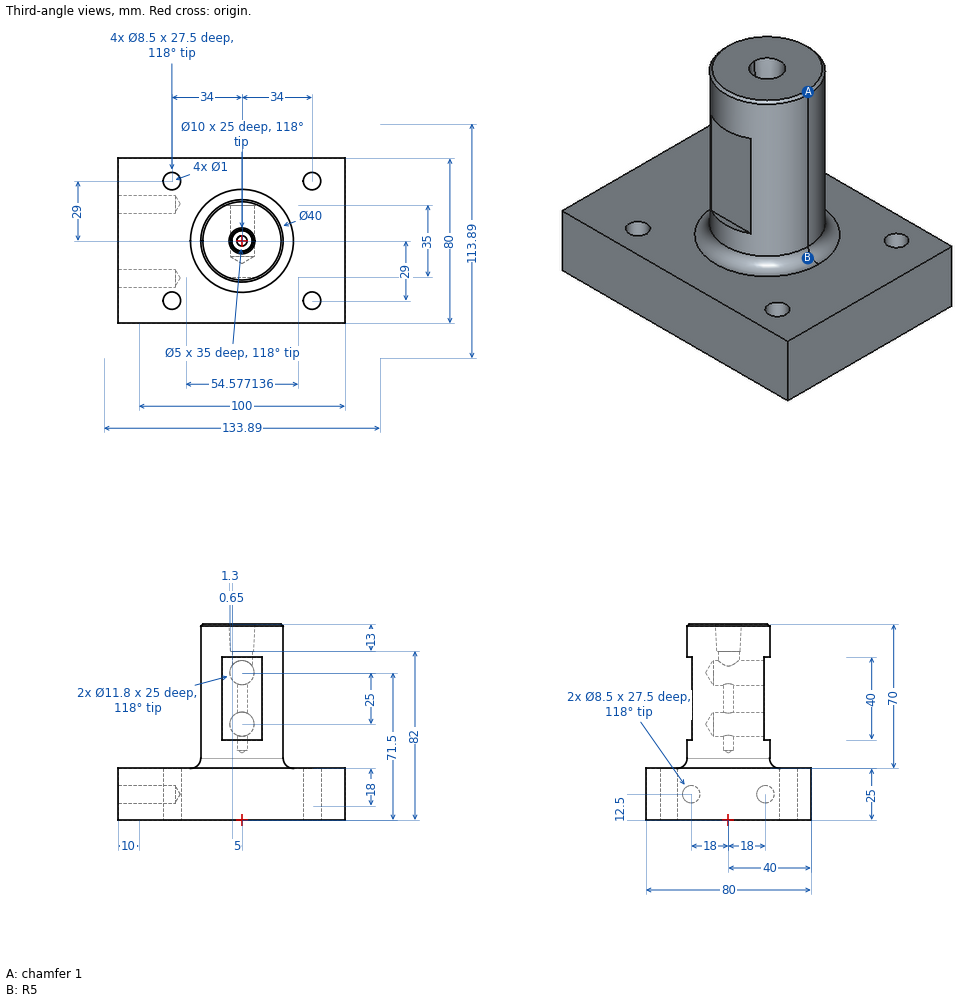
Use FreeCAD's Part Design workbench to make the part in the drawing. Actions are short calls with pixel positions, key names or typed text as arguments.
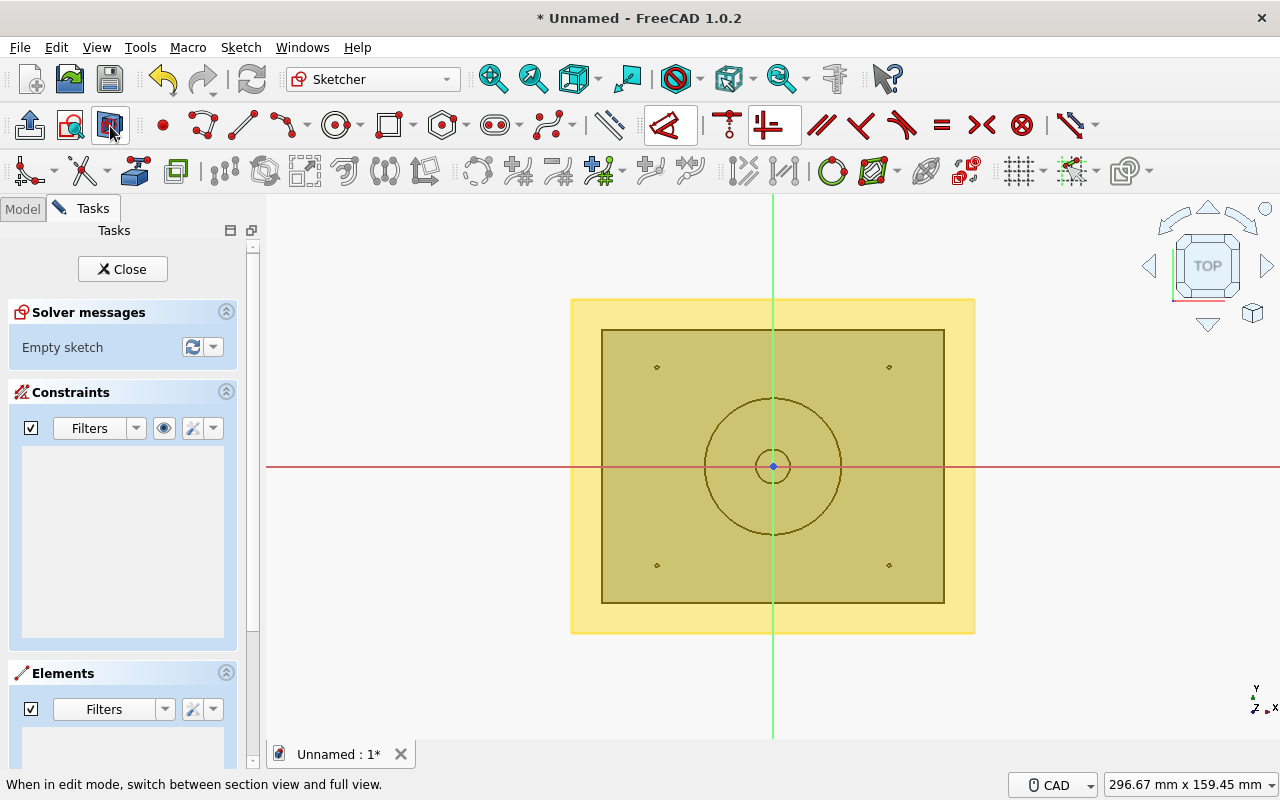
click(416, 126)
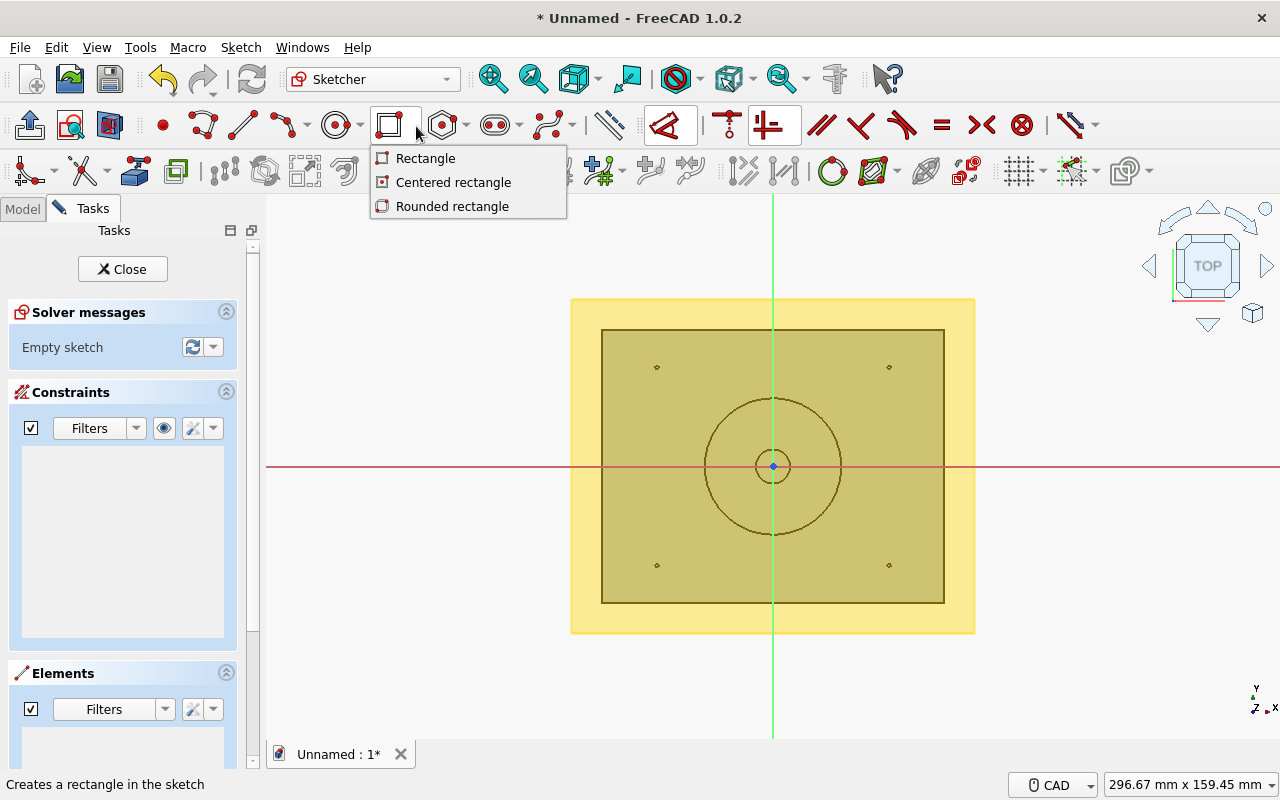
click(468, 182)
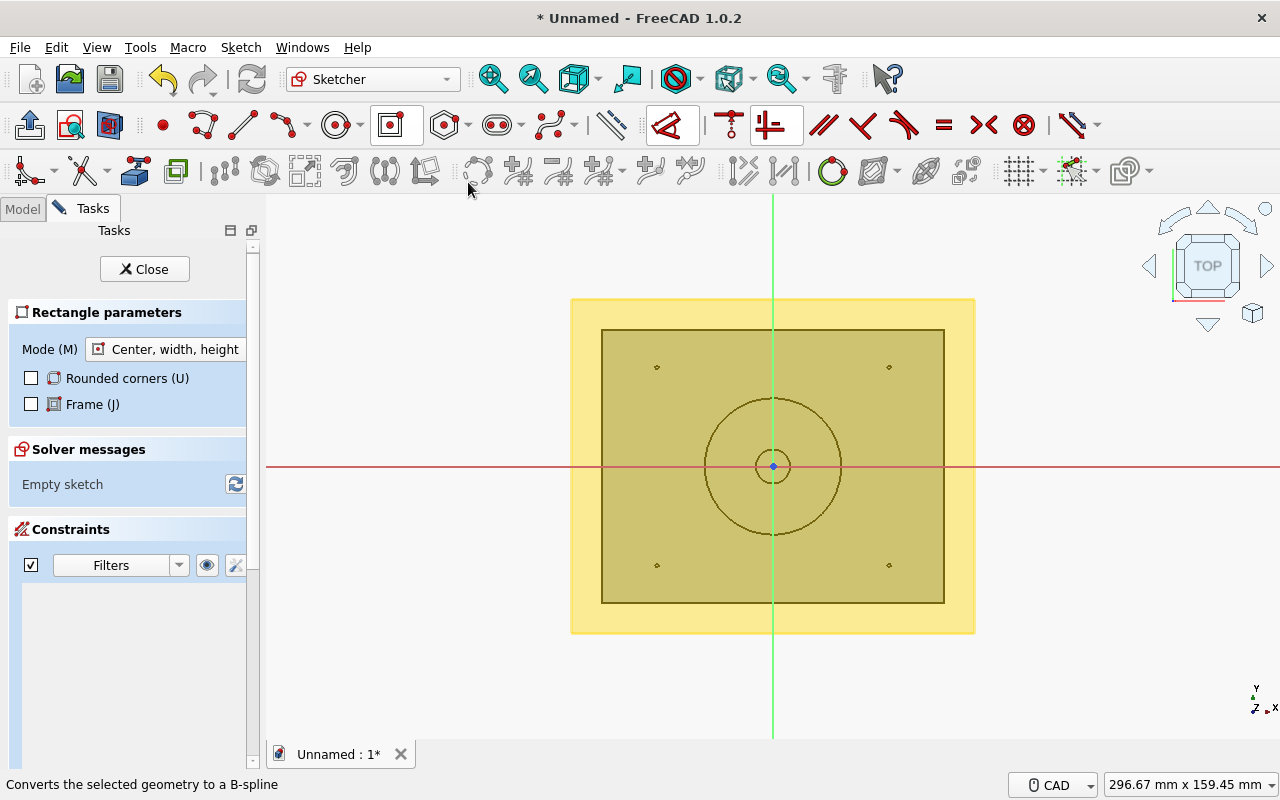
click(773, 466)
click(1002, 272)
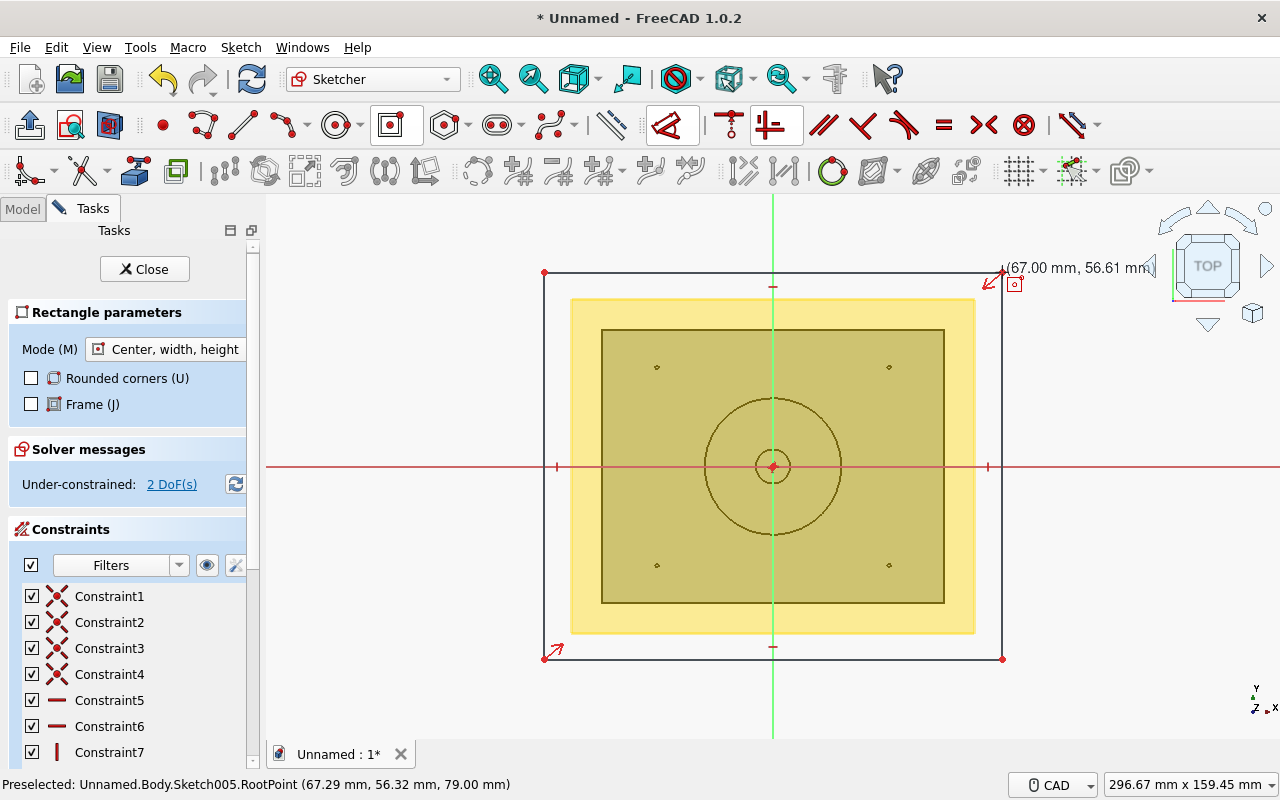
click(773, 466)
click(866, 407)
key(Escape)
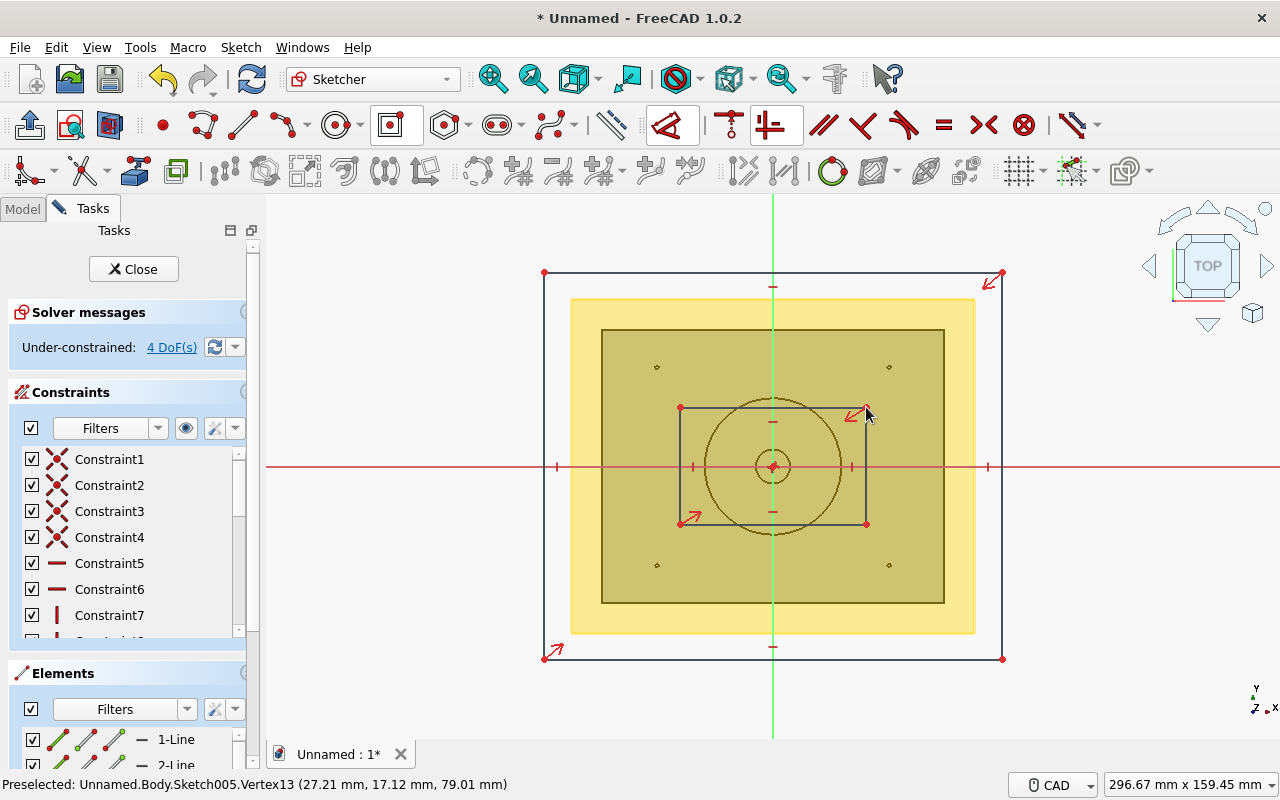
click(866, 490)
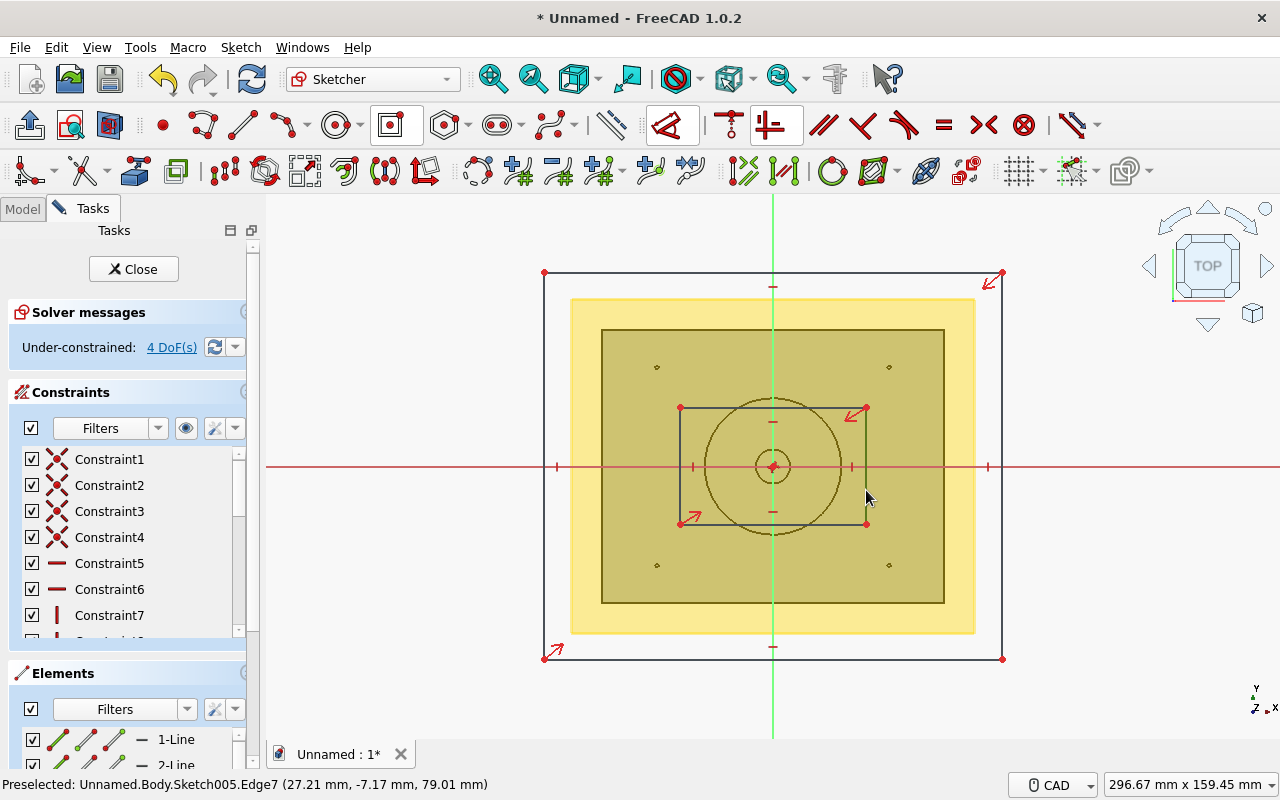
key(i)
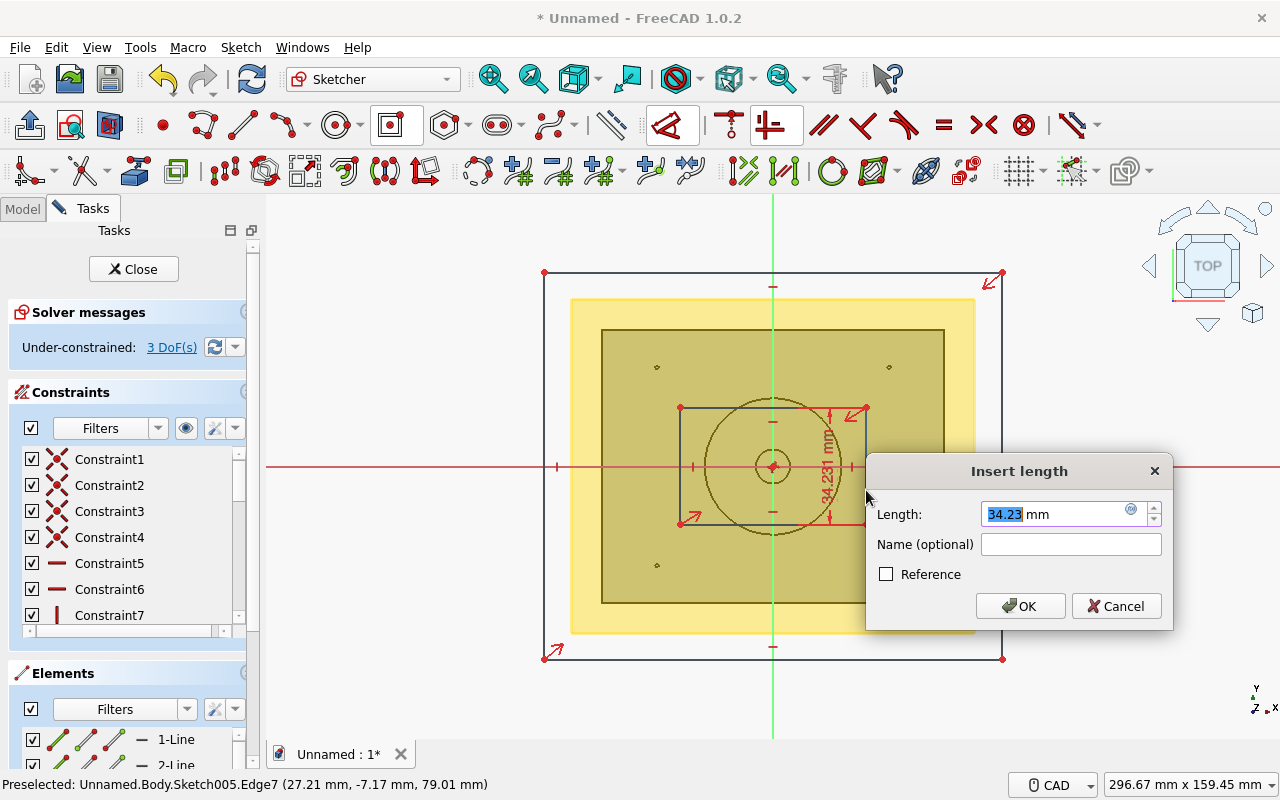
text(35)
key(Return)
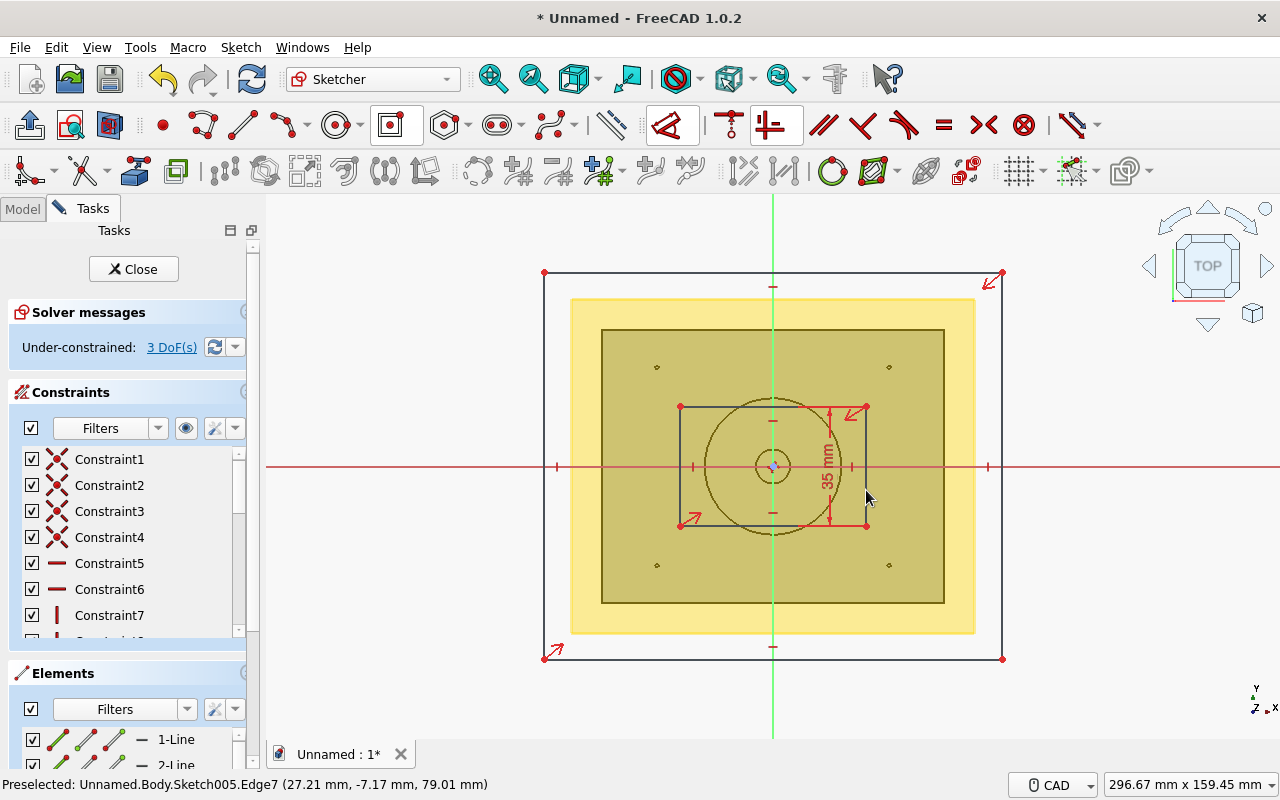
click(681, 660)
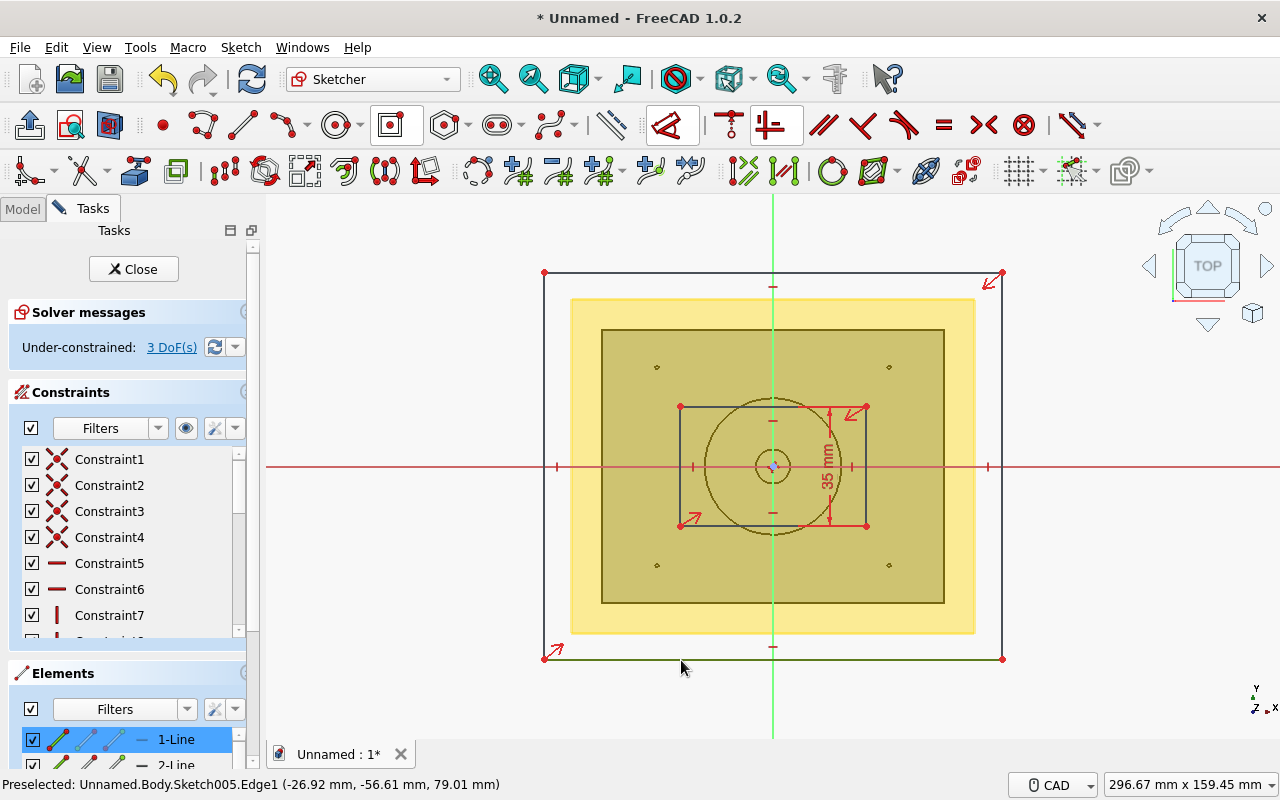
key(l)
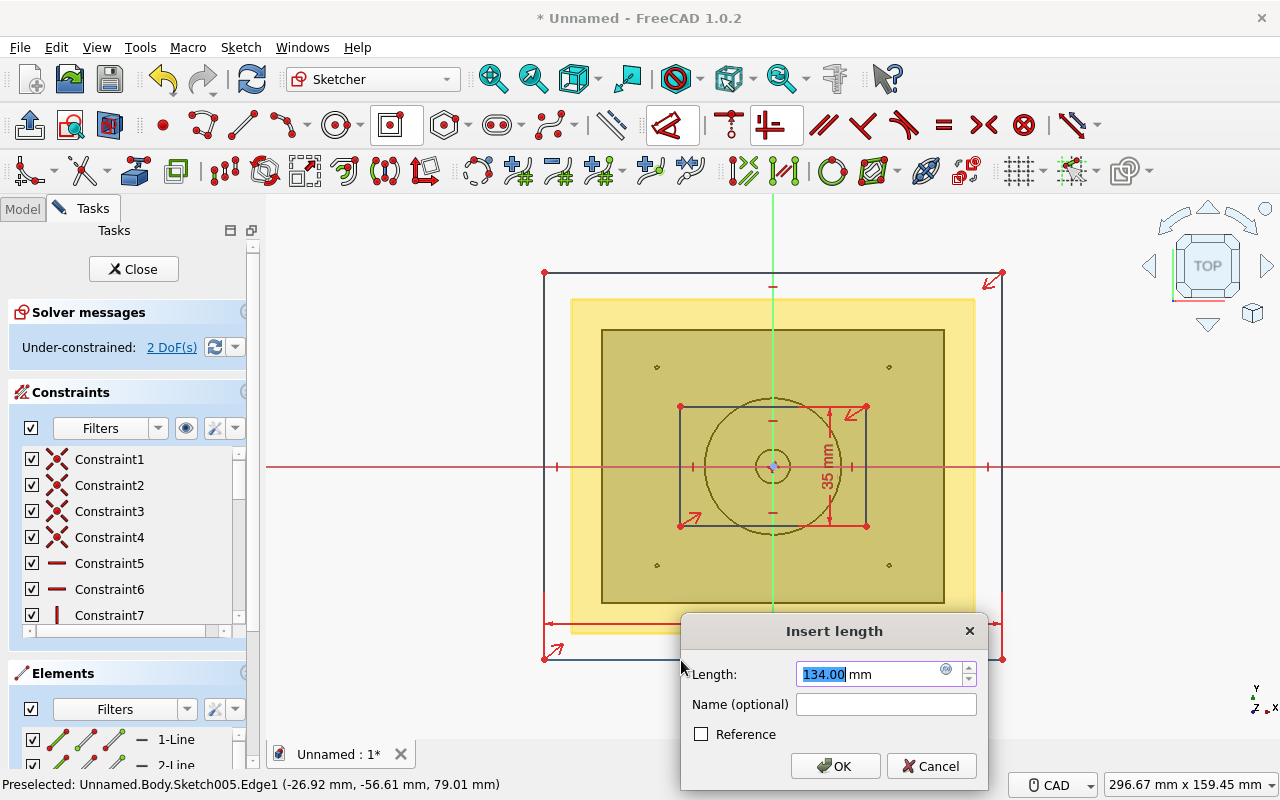
text(133.89)
key(Return)